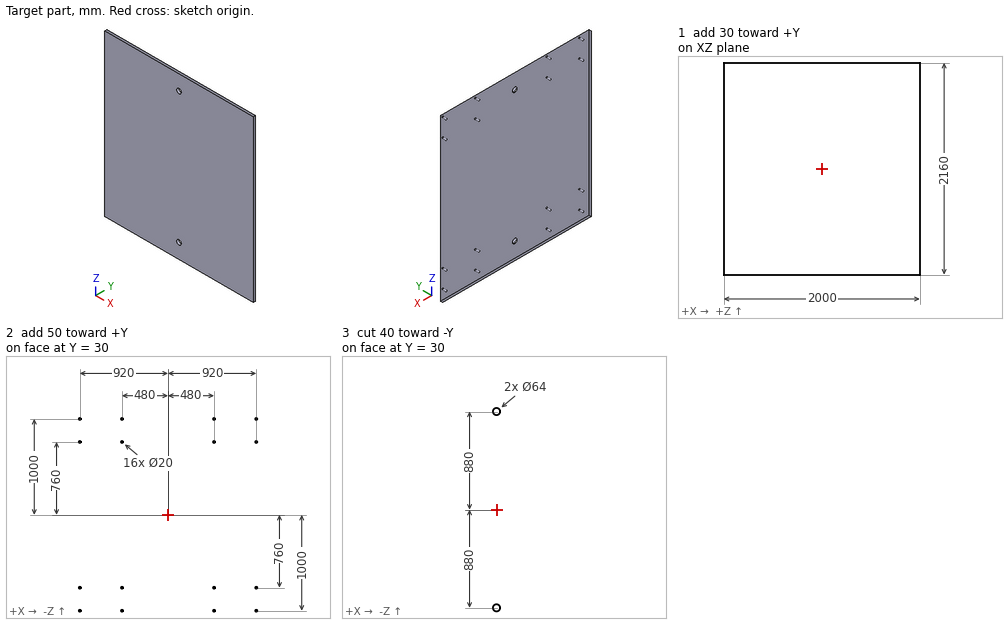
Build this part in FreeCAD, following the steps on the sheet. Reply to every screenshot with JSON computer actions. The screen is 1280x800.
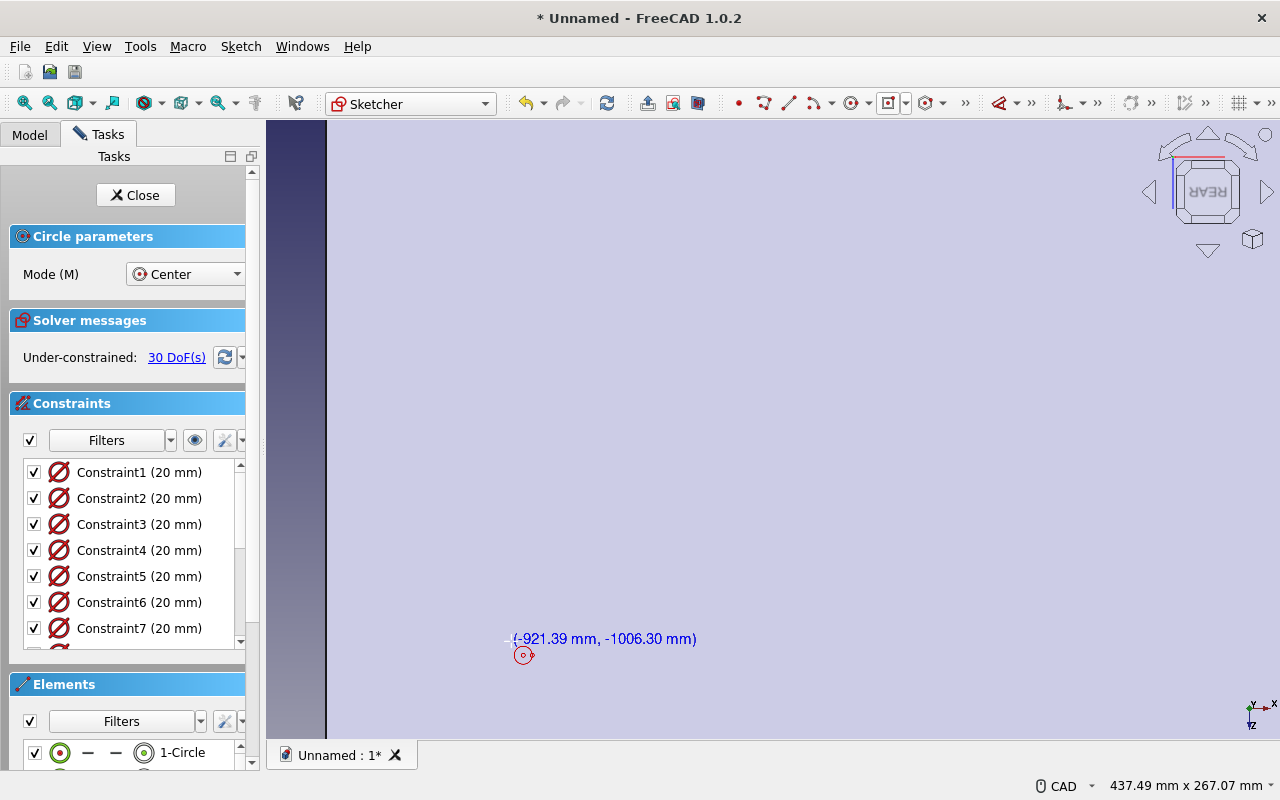
{"action": "scroll", "coordinate": [511, 641], "scroll_direction": "down", "scroll_amount": 12}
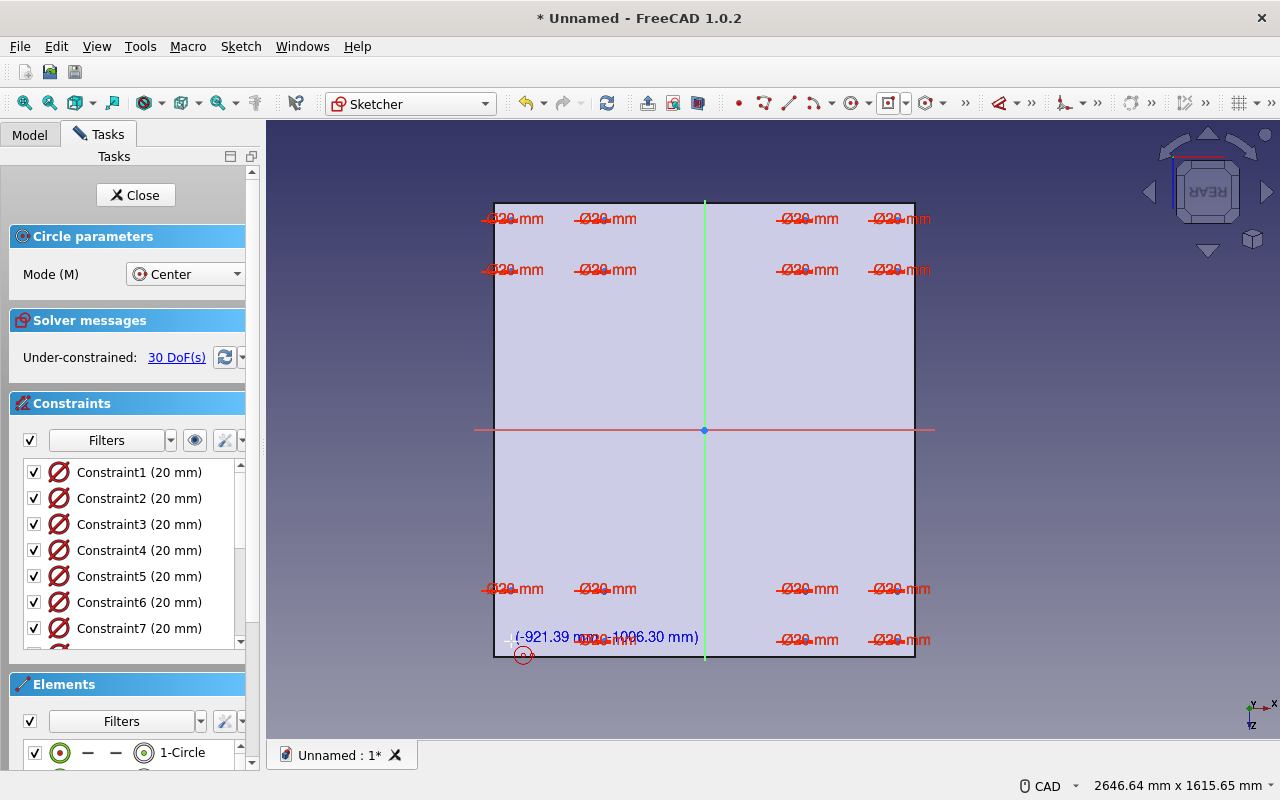
{"action": "left_click", "coordinate": [511, 641]}
{"action": "mouse_move", "coordinate": [513, 639]}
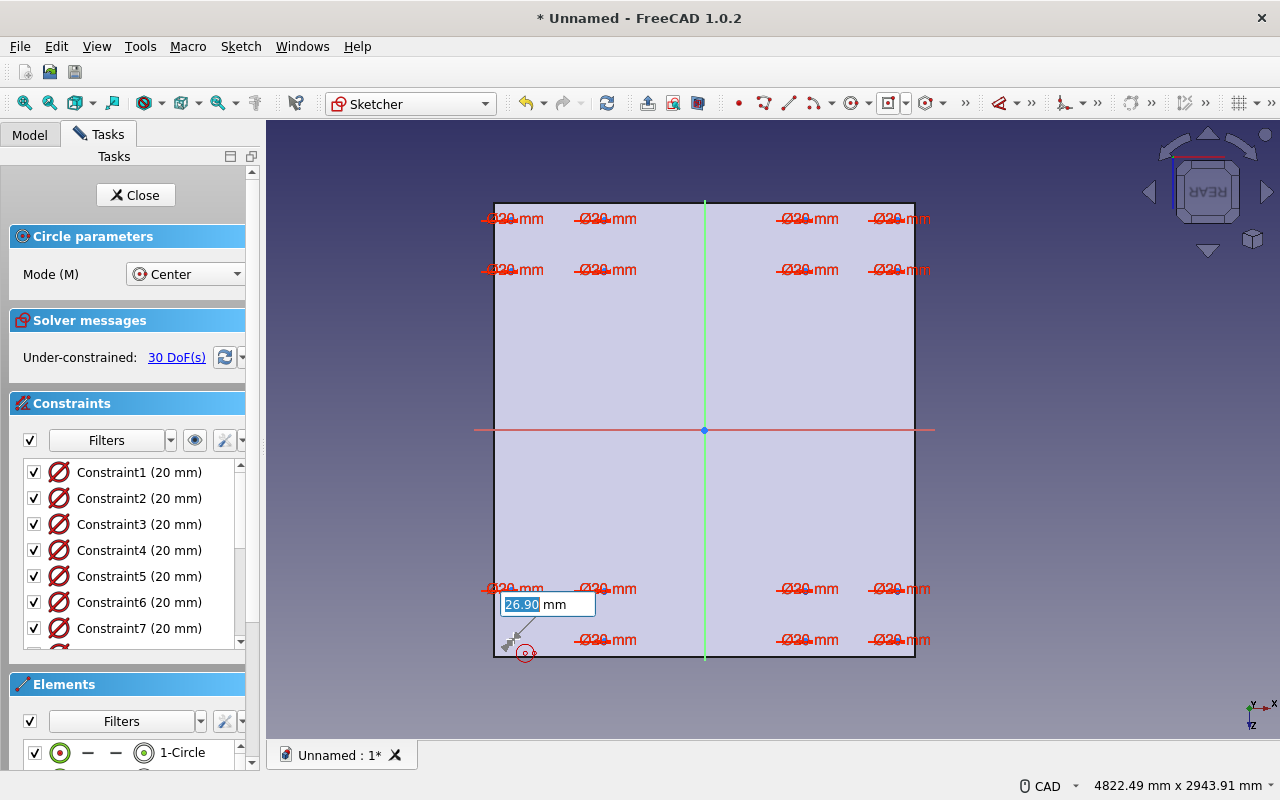
{"action": "type", "text": "20"}
{"action": "key", "text": "Return"}
{"action": "key", "text": "Escape"}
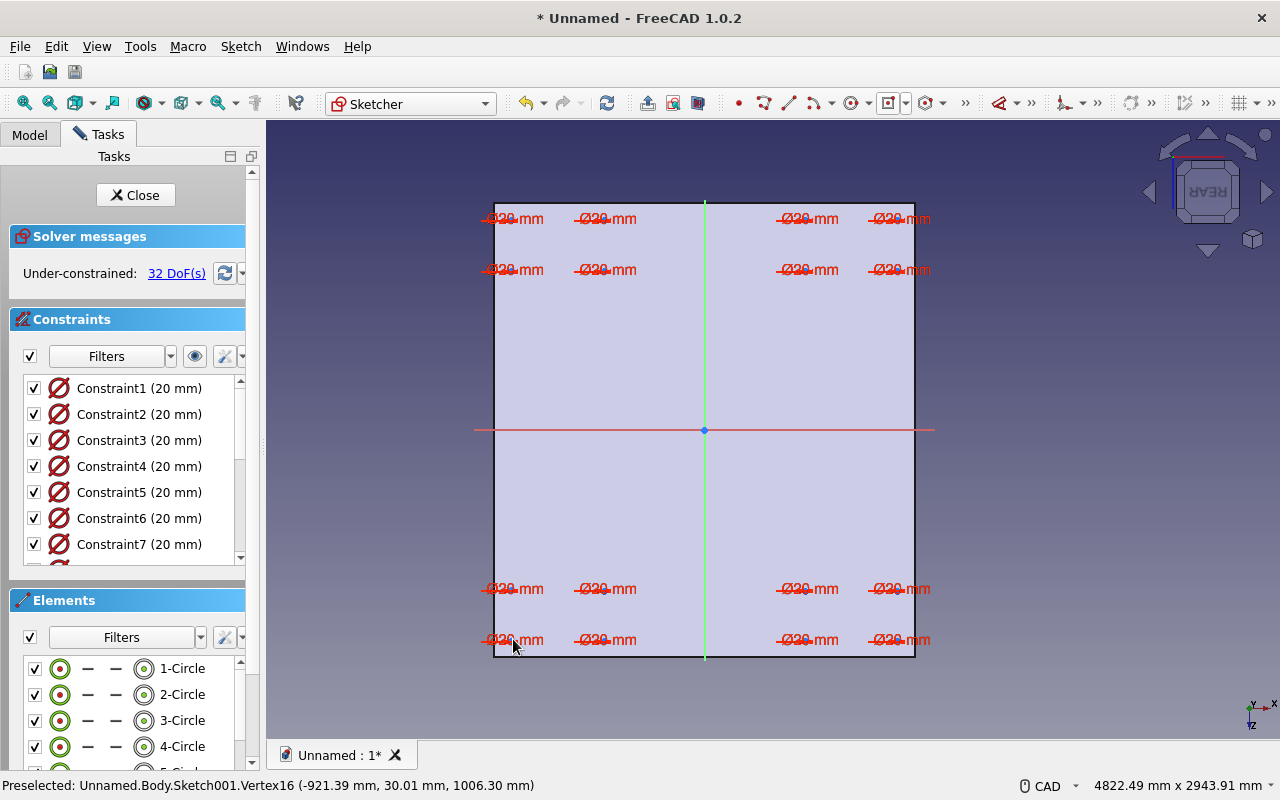
{"action": "left_click", "coordinate": [511, 221]}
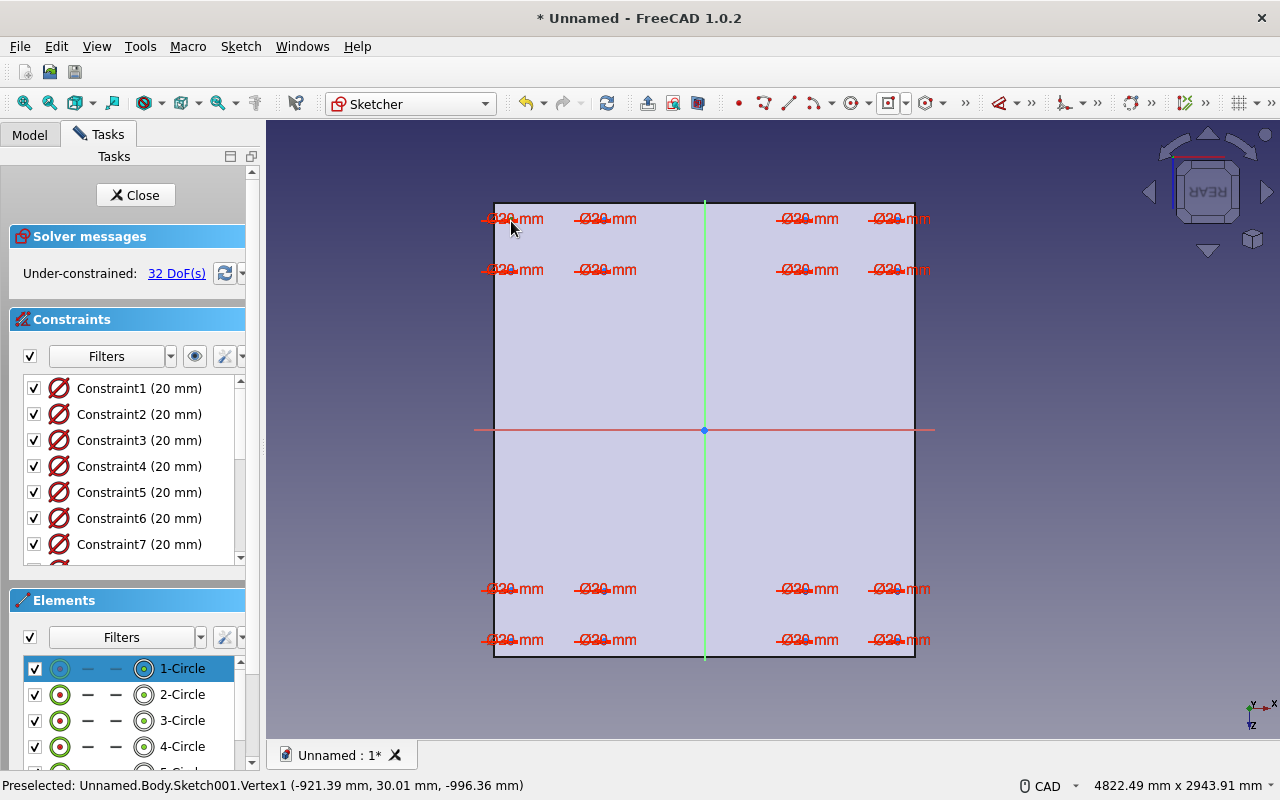
{"action": "left_click", "coordinate": [511, 272]}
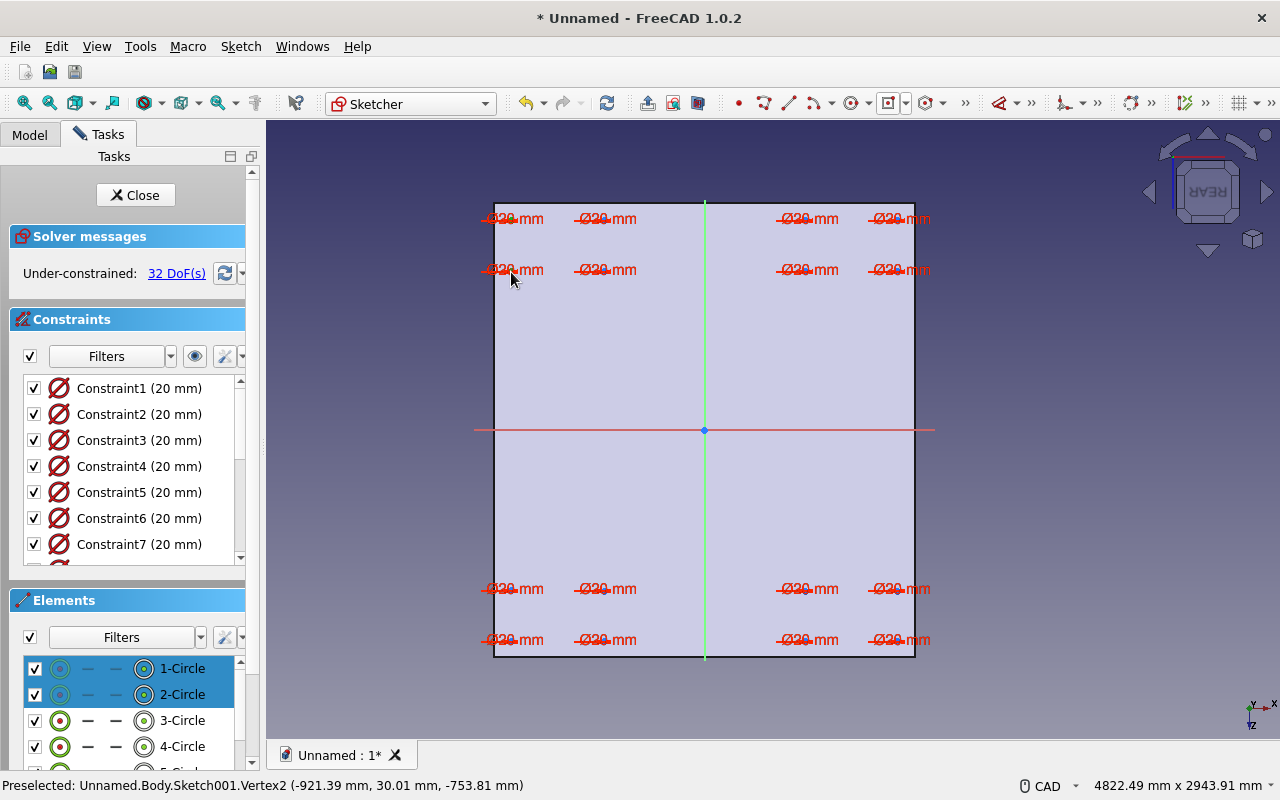
{"action": "key", "text": "v"}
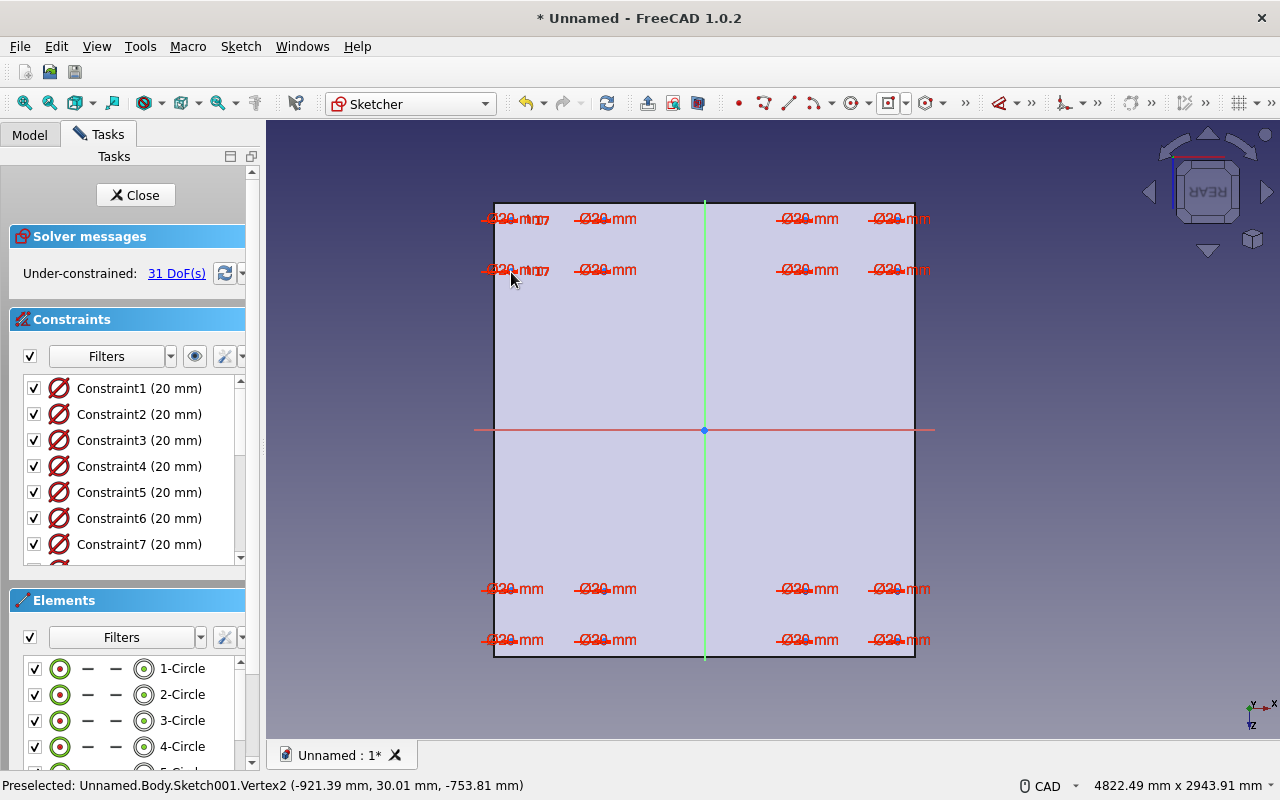
{"action": "left_click", "coordinate": [511, 221]}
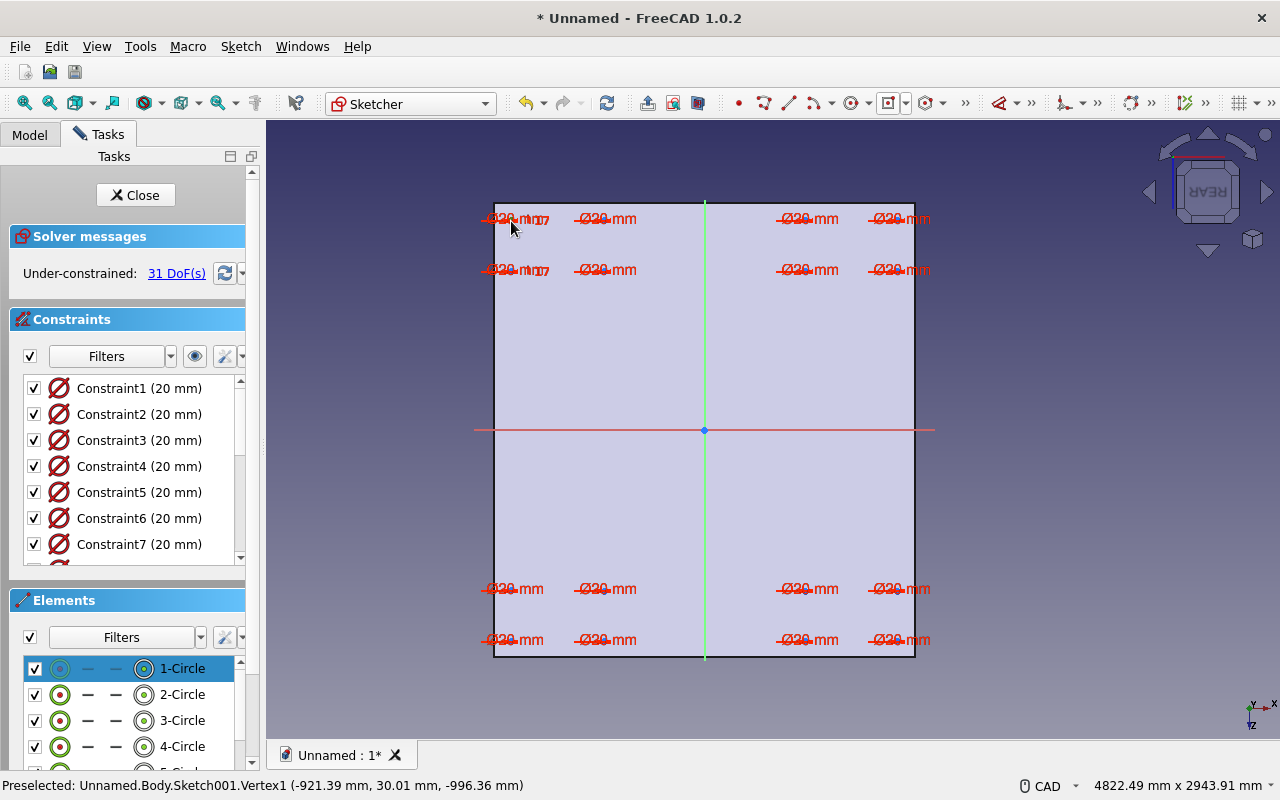
{"action": "left_click", "coordinate": [604, 221]}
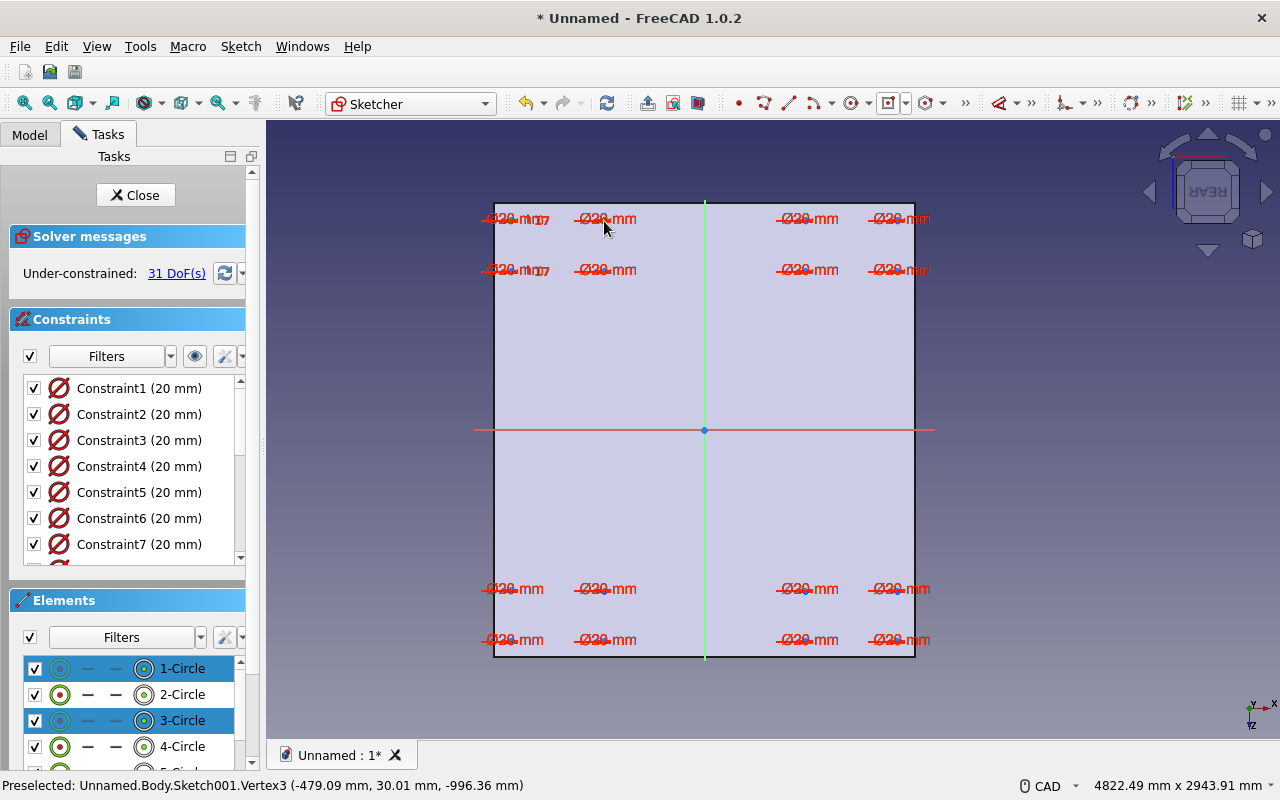
{"action": "key", "text": "h"}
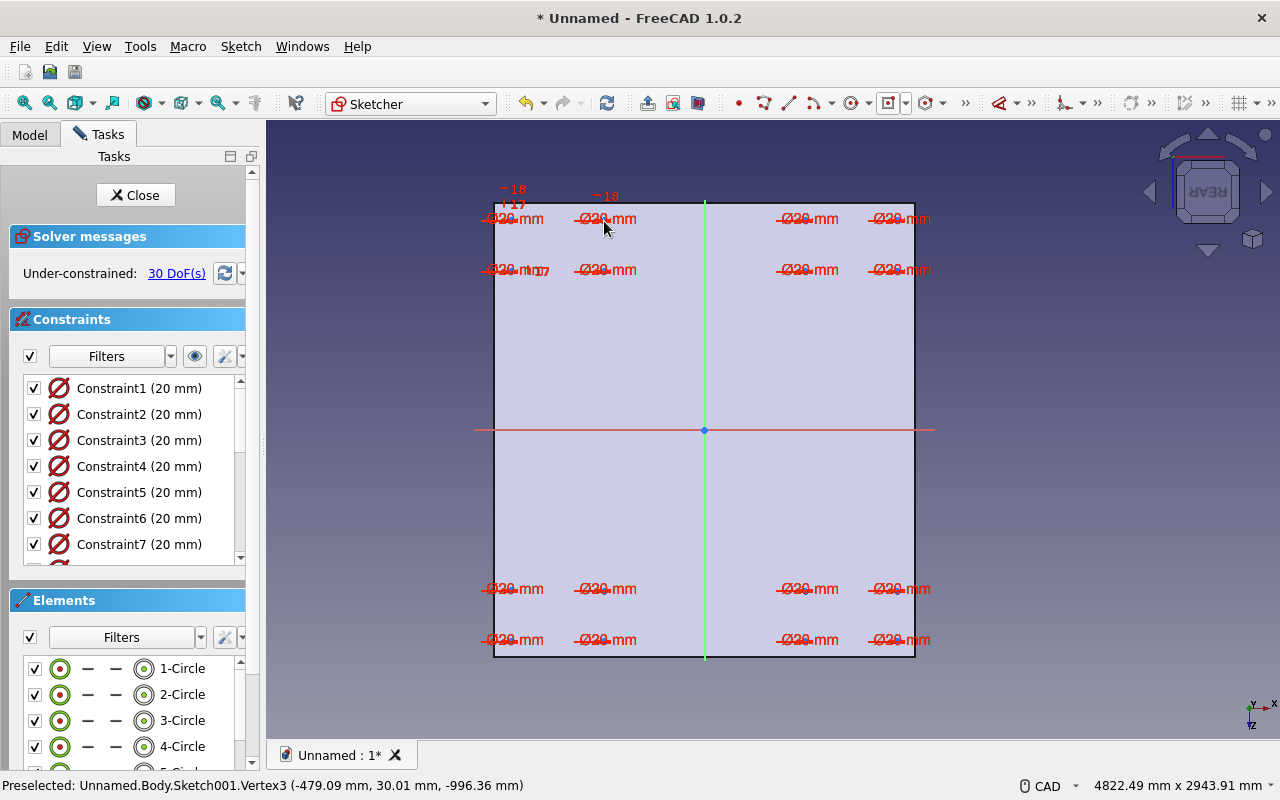
{"action": "left_click", "coordinate": [604, 221]}